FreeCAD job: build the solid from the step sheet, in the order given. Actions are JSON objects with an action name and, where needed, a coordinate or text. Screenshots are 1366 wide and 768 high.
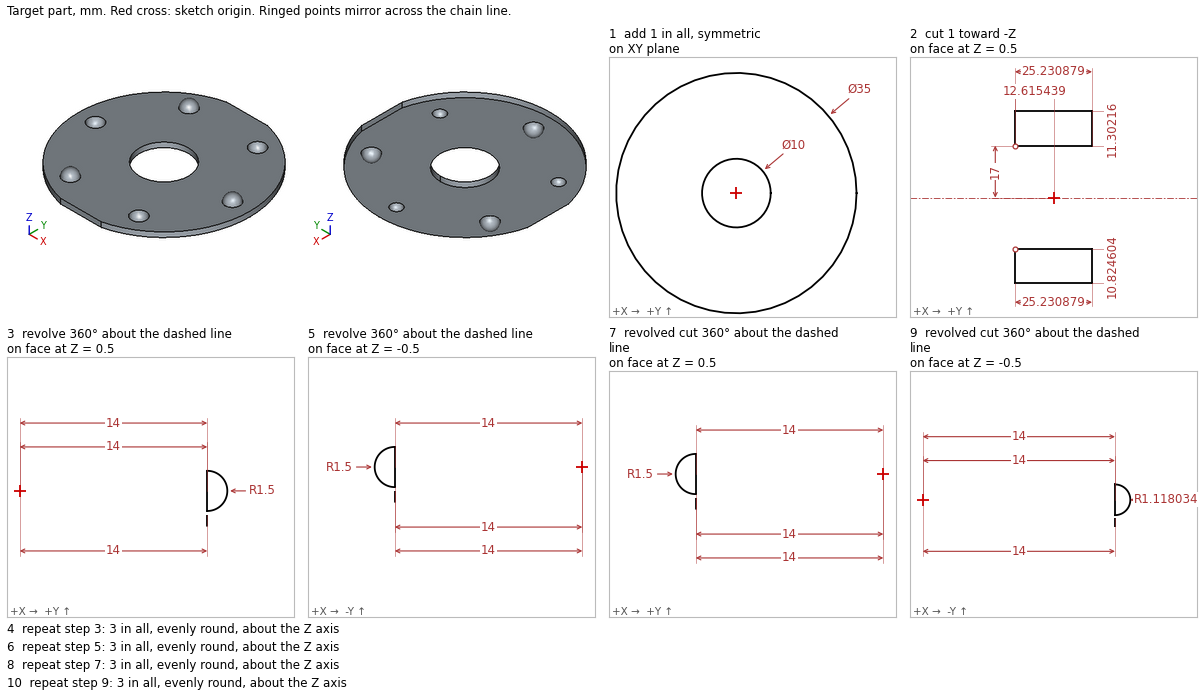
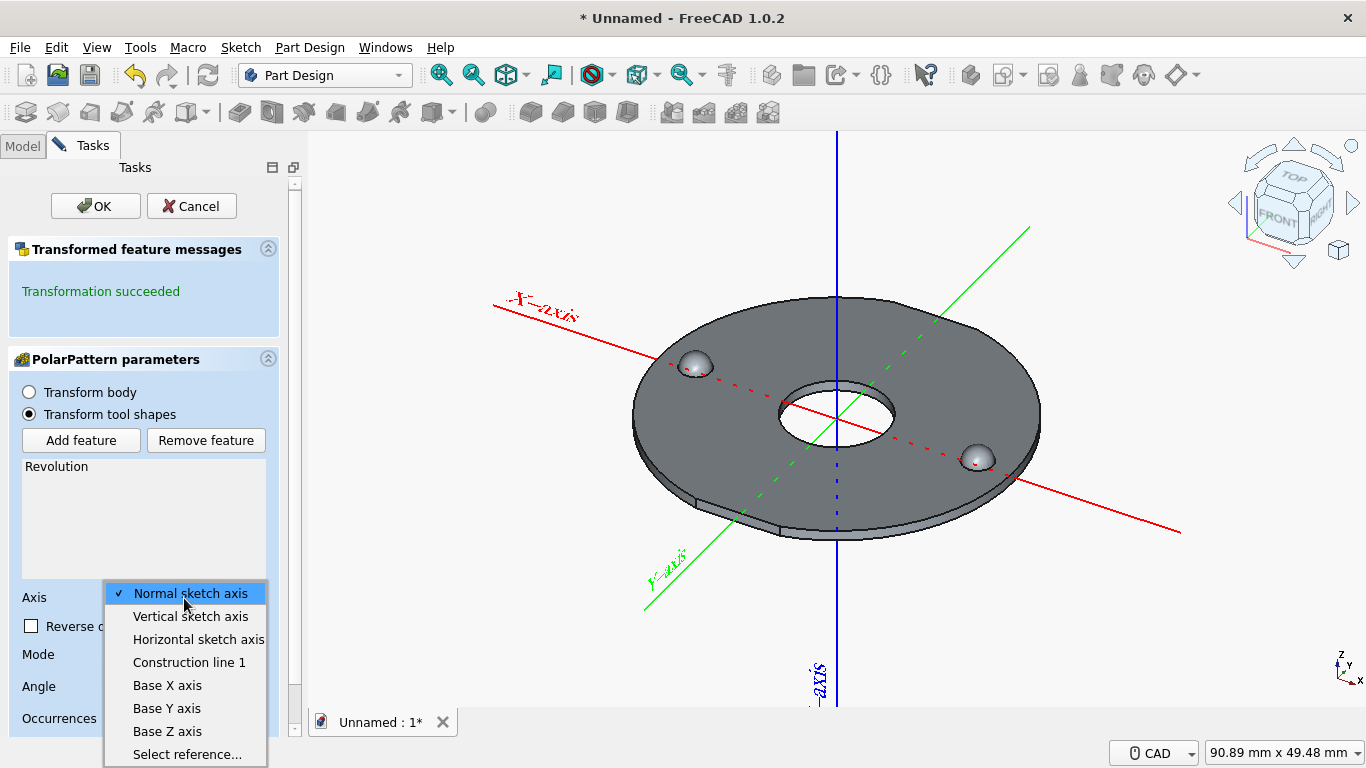
{"action": "left_click", "coordinate": [184, 732]}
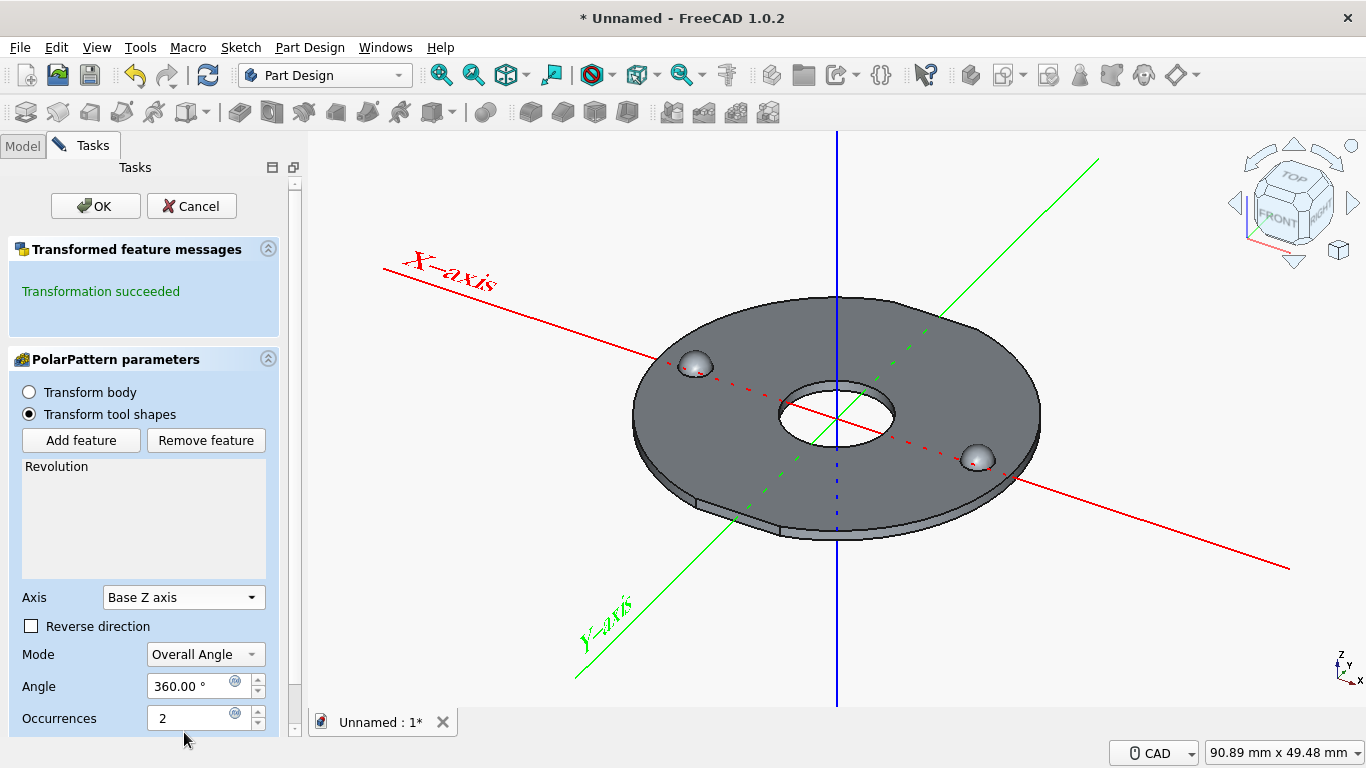
{"action": "triple_click", "coordinate": [198, 718]}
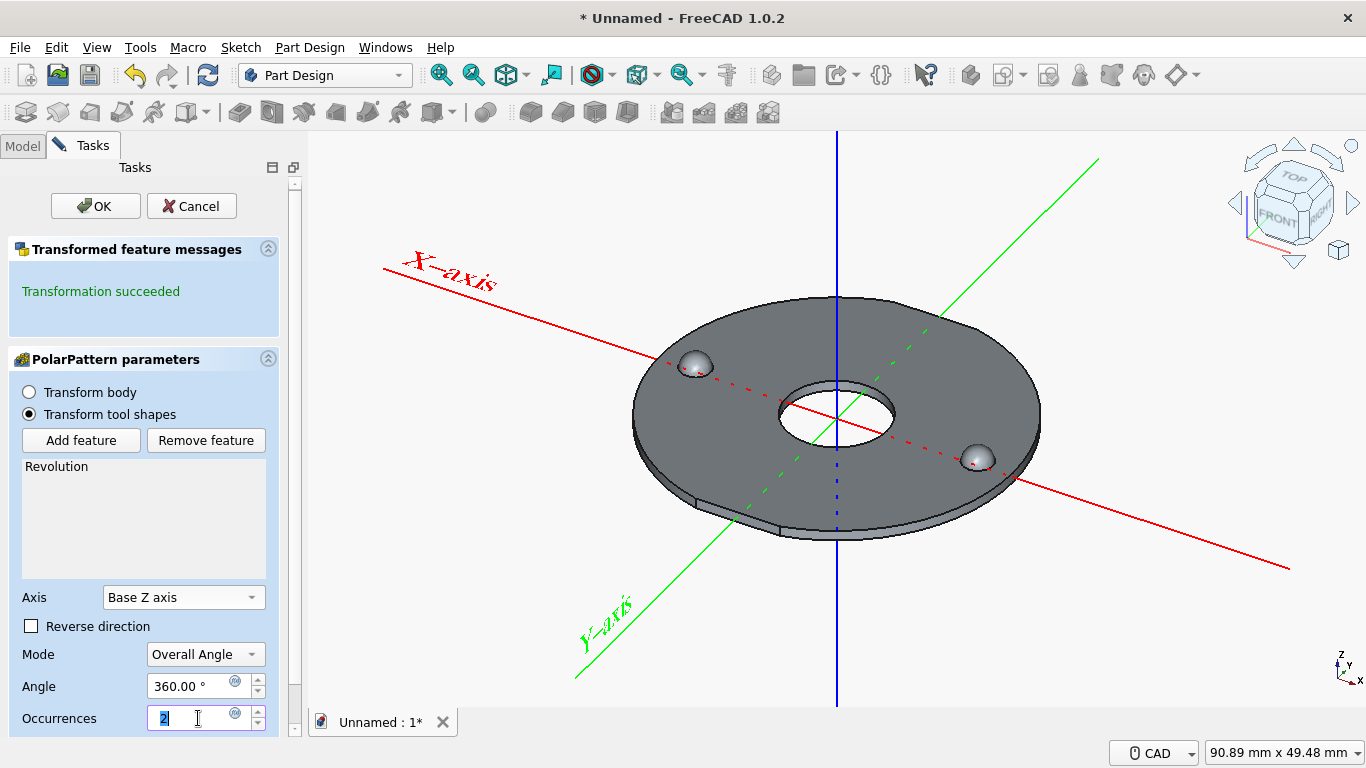
{"action": "type", "text": "3"}
{"action": "key", "text": "Tab"}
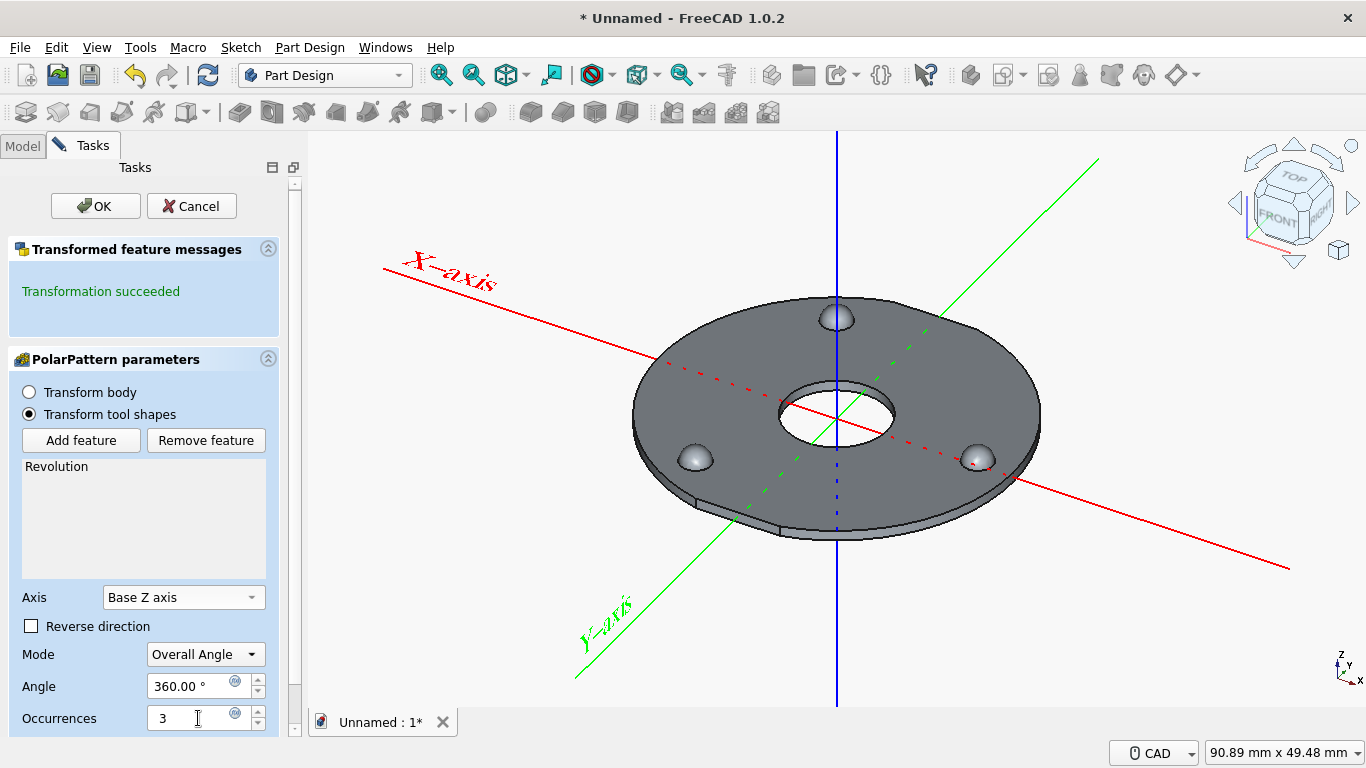
{"action": "left_click", "coordinate": [96, 206]}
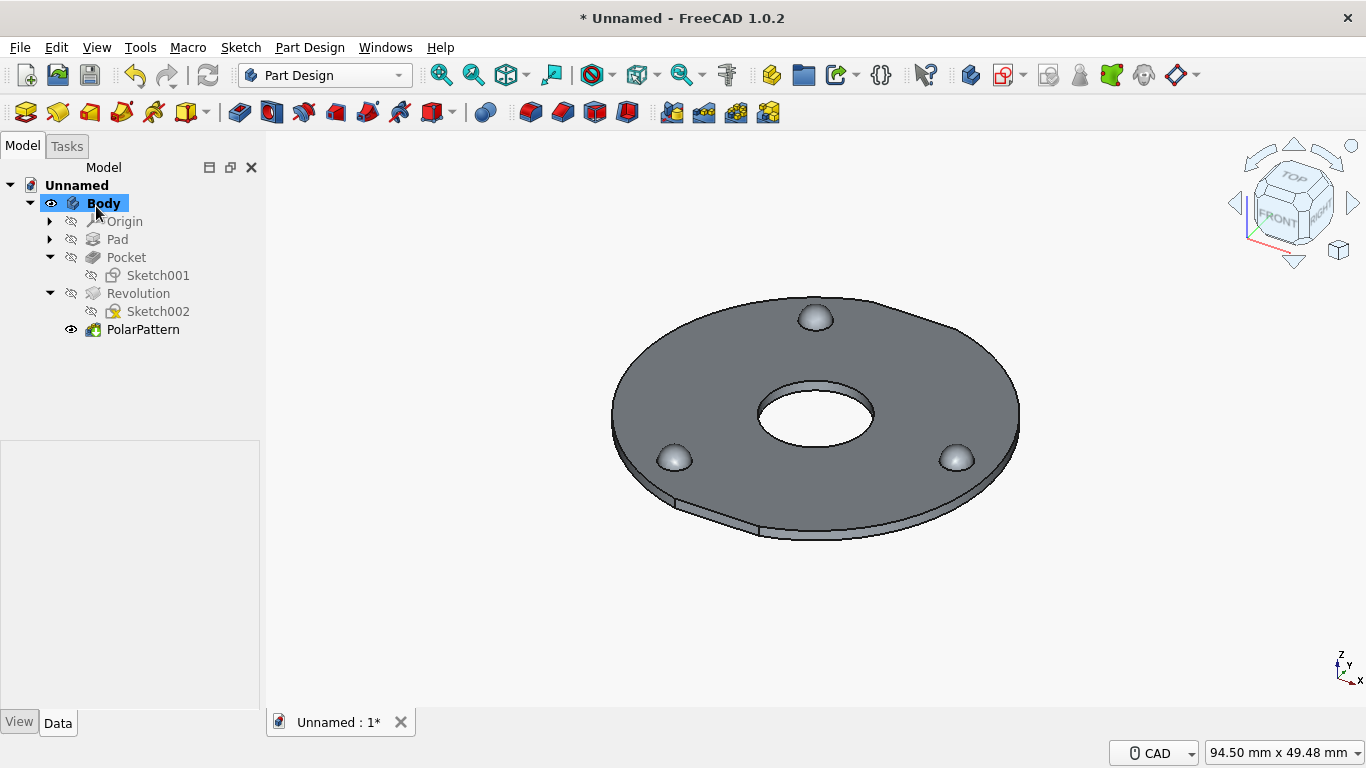
{"action": "key", "text": "5"}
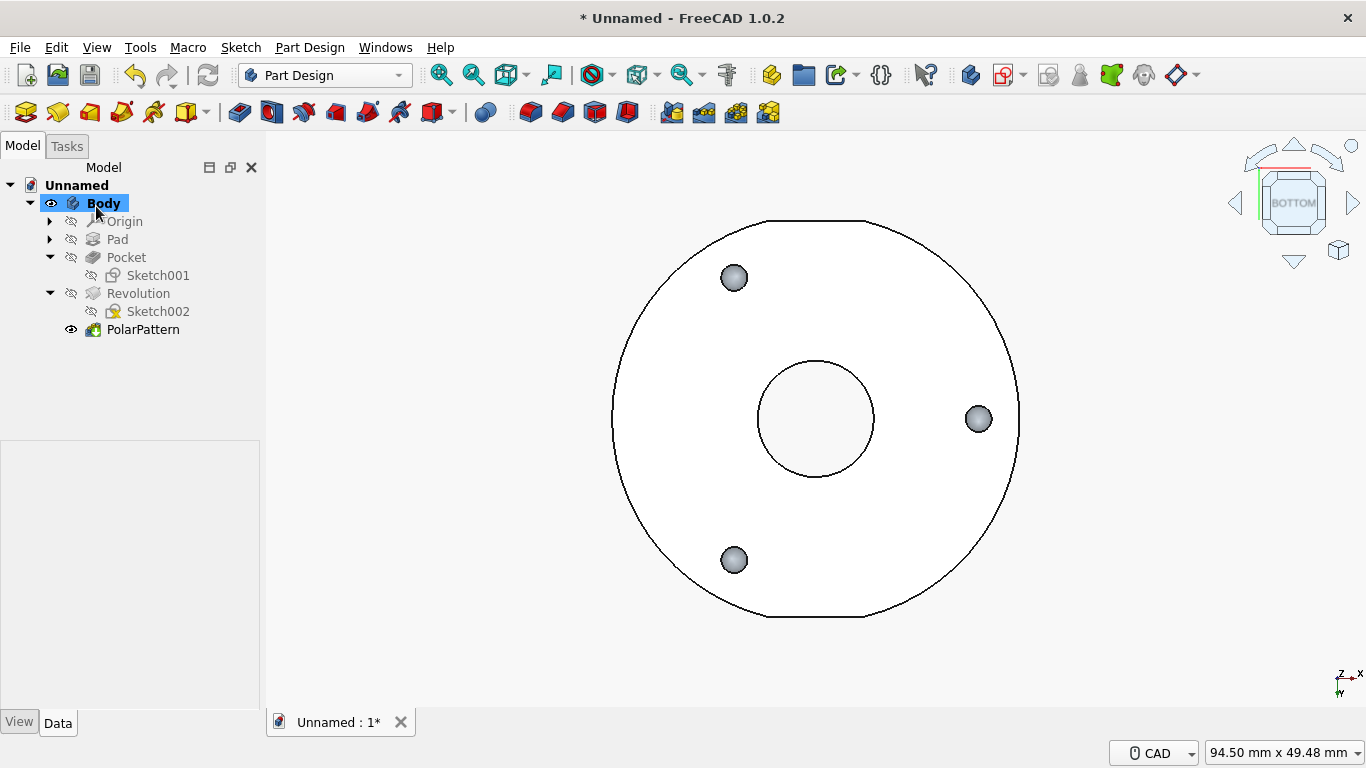
{"action": "left_click", "coordinate": [699, 361]}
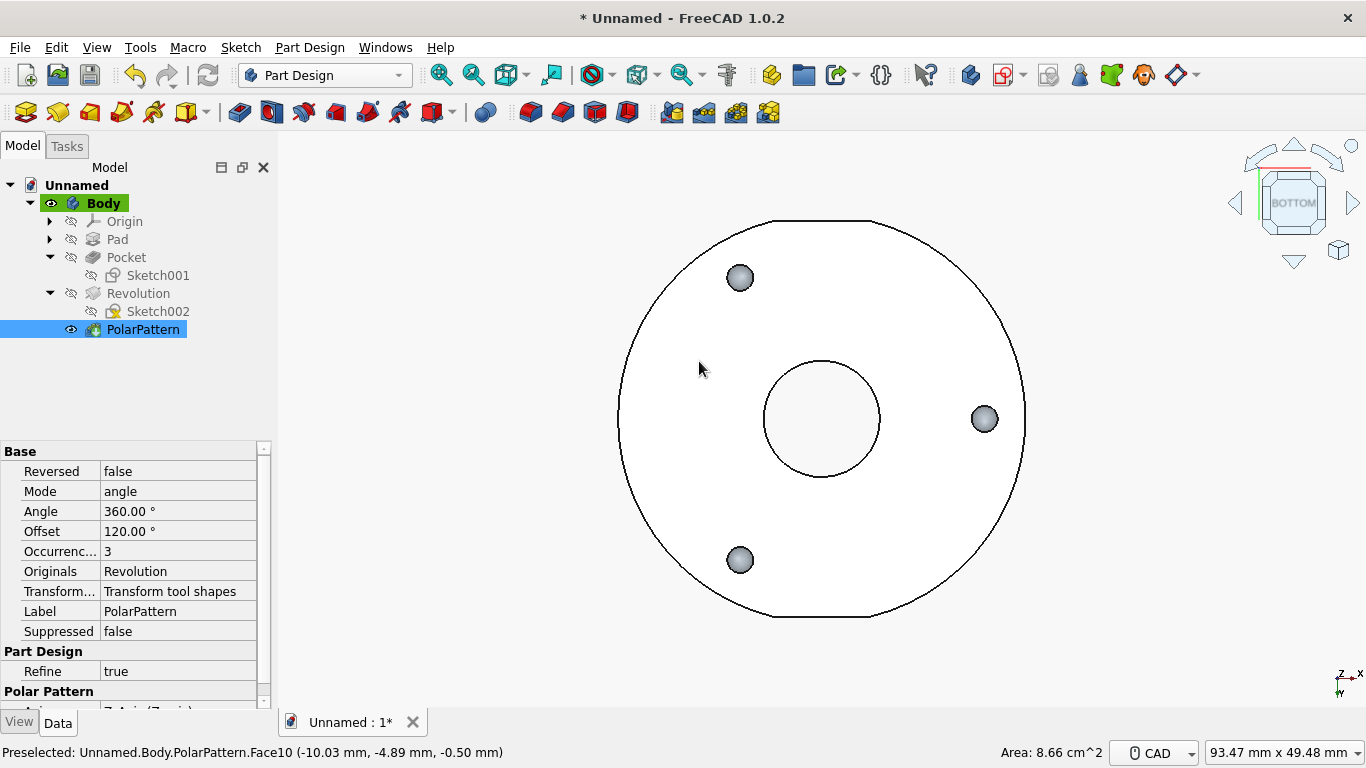
{"action": "left_click", "coordinate": [1004, 76]}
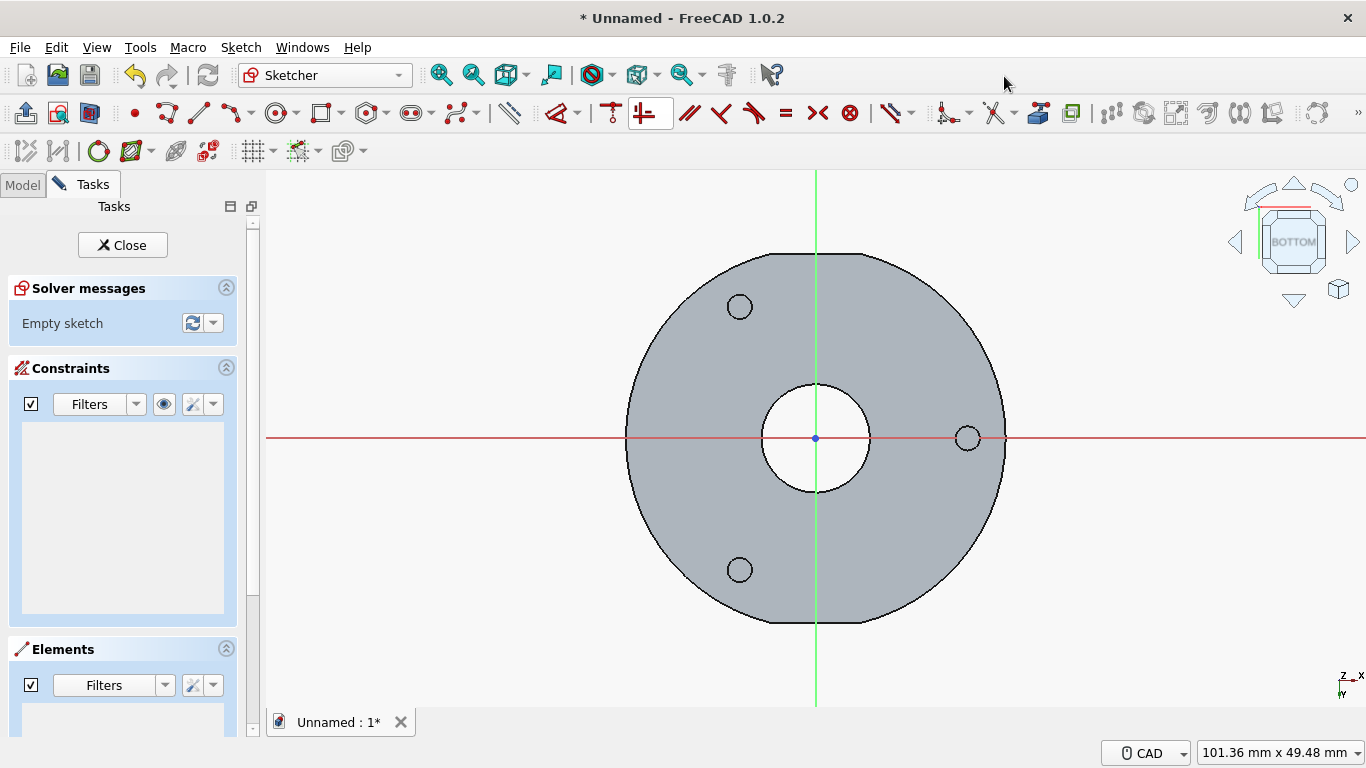
{"action": "left_click", "coordinate": [90, 114]}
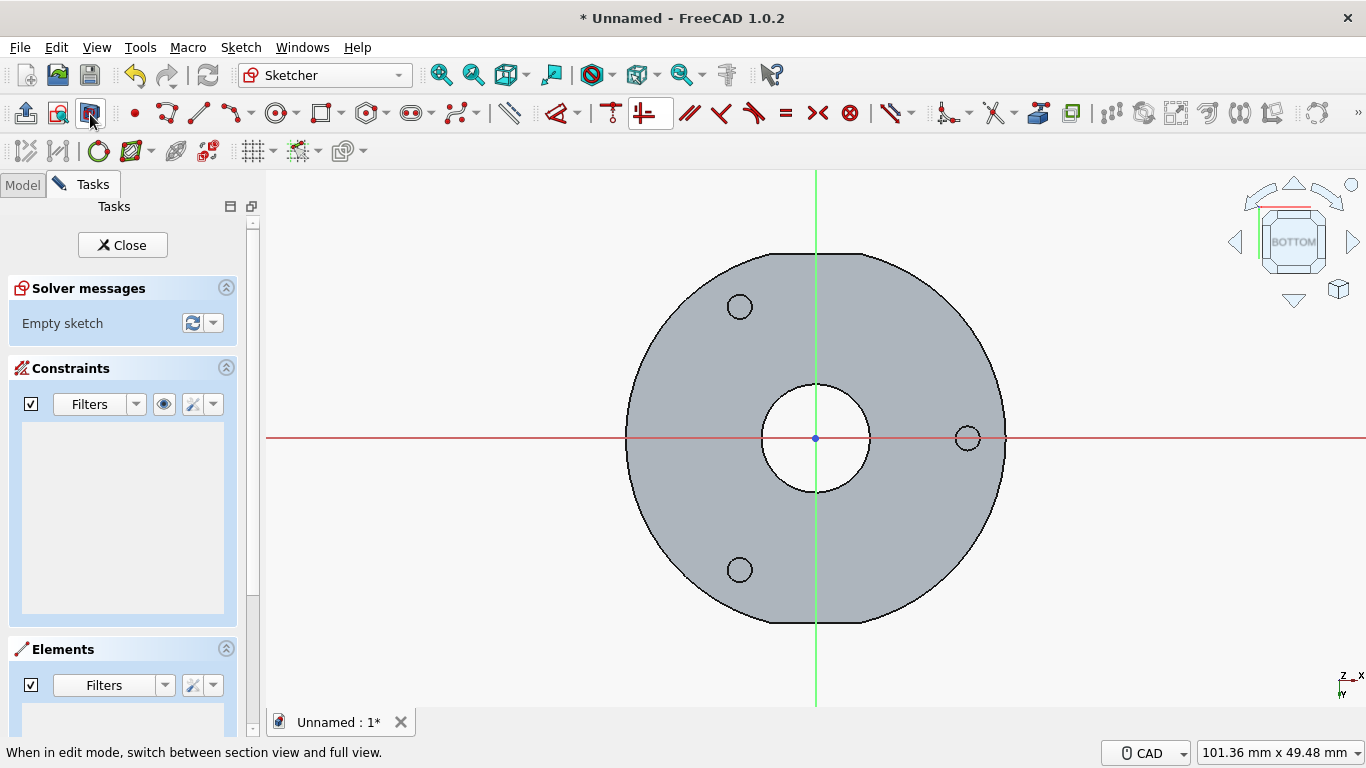
{"action": "scroll", "coordinate": [641, 446], "scroll_direction": "up", "scroll_amount": 10}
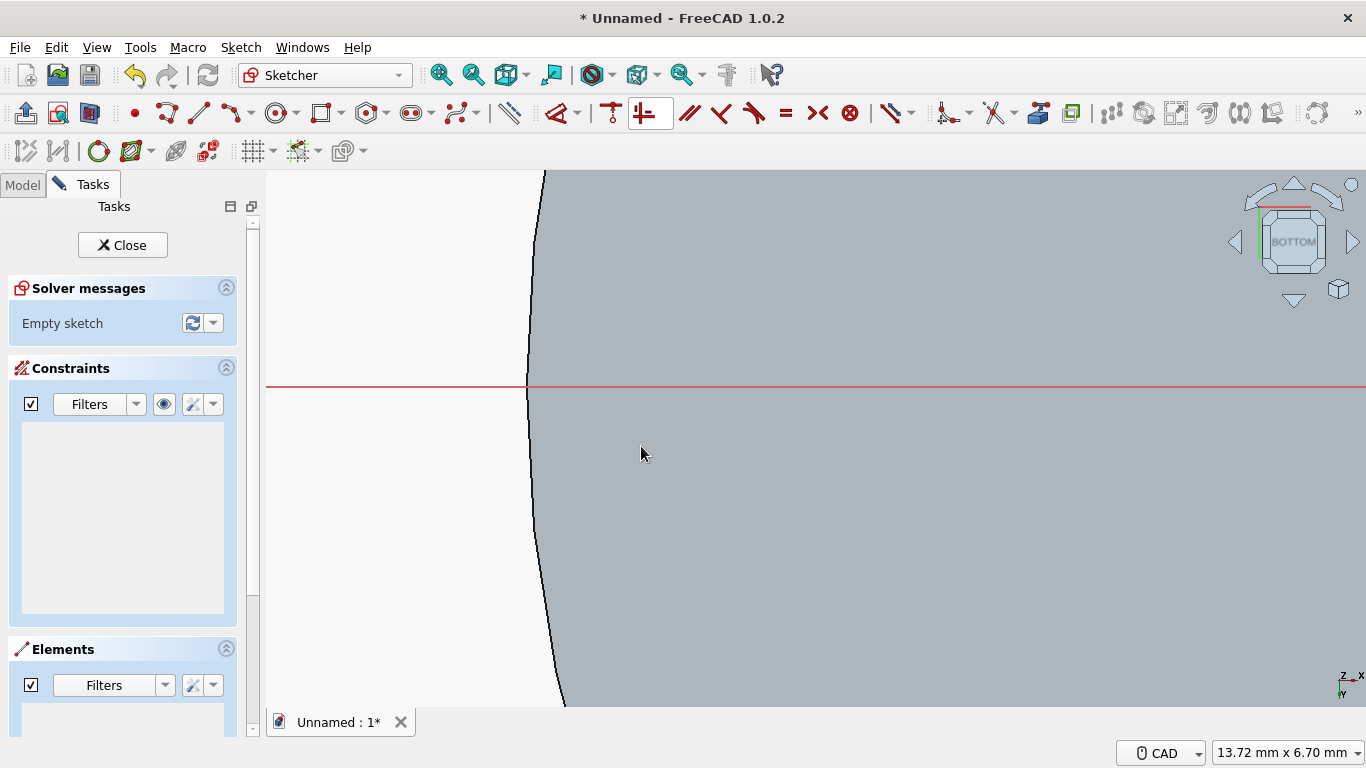
{"action": "key", "text": "g l"}